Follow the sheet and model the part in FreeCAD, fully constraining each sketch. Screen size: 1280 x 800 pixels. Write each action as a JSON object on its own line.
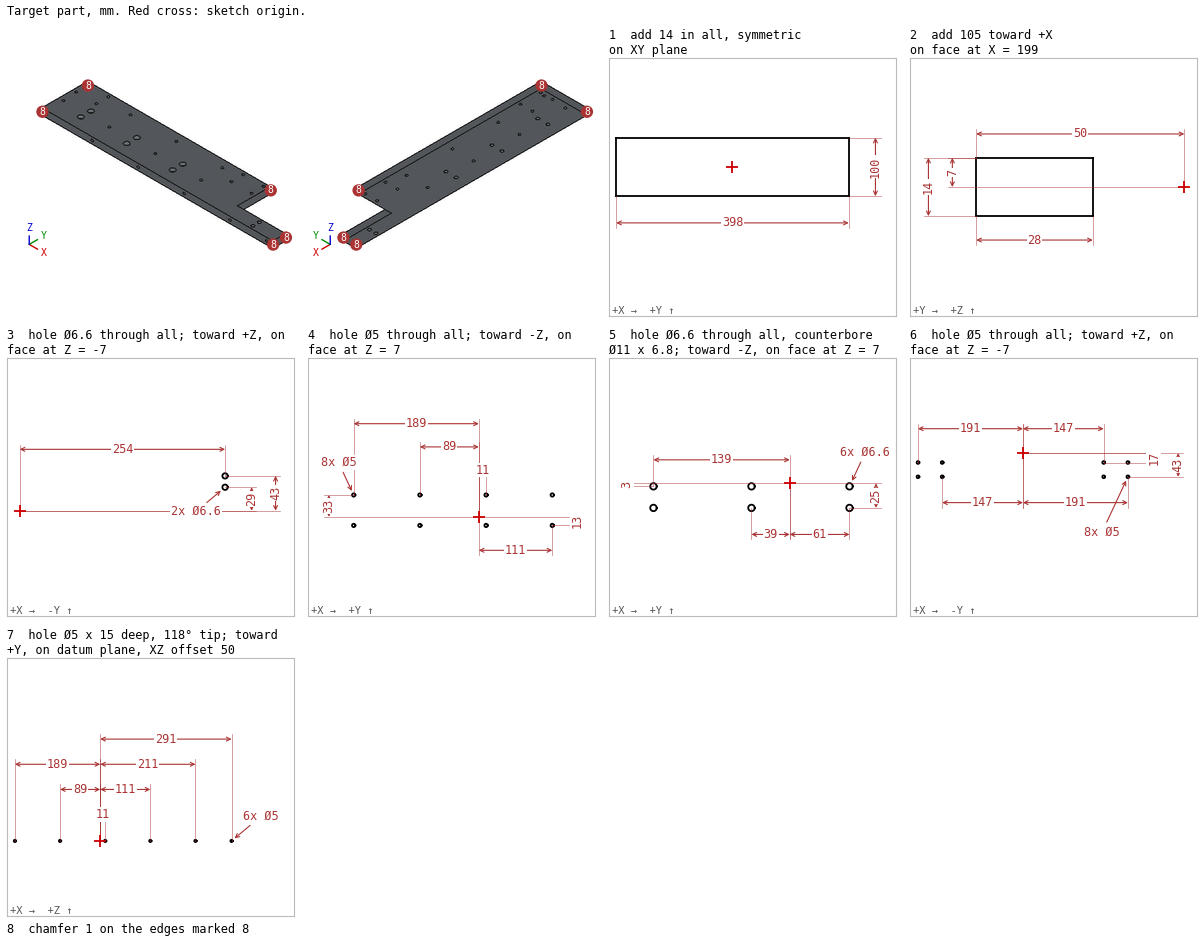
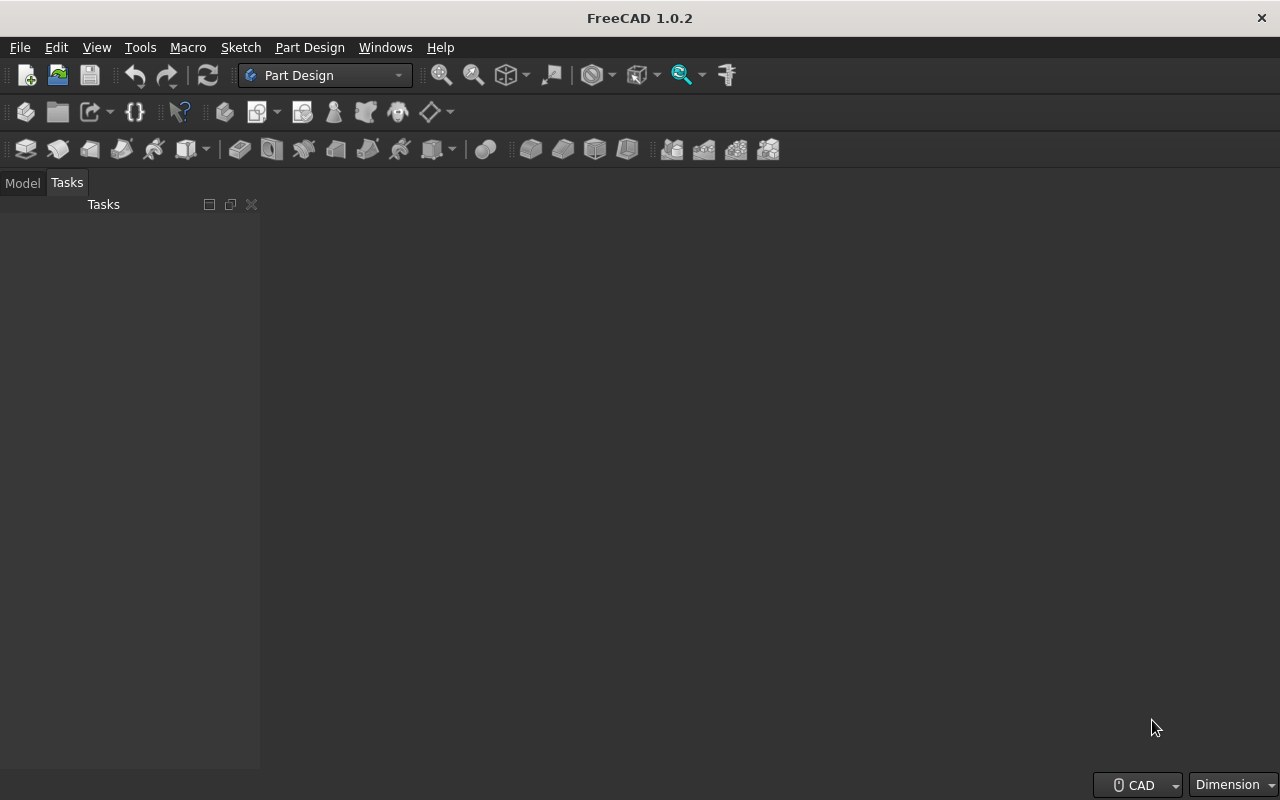
{"action": "key", "text": "ctrl+n"}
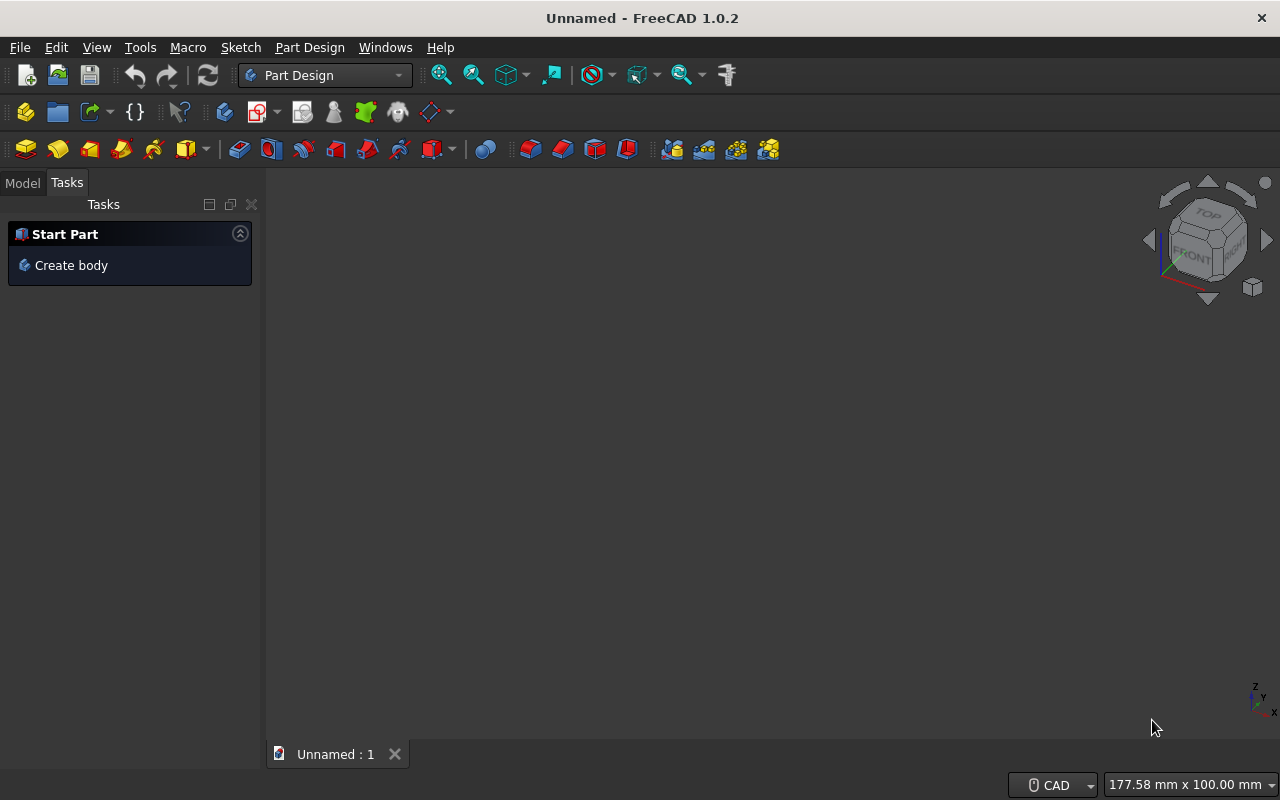
{"action": "left_click", "coordinate": [258, 112]}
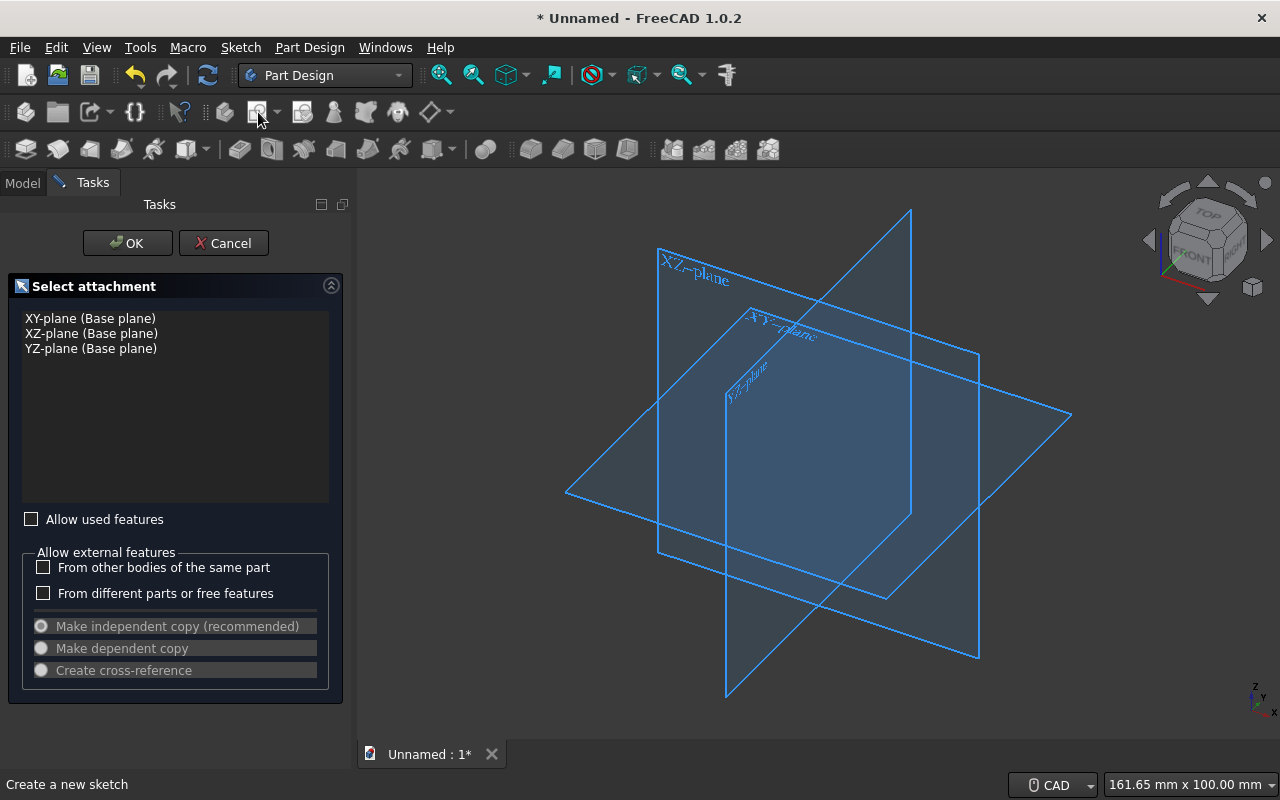
{"action": "left_click", "coordinate": [82, 318]}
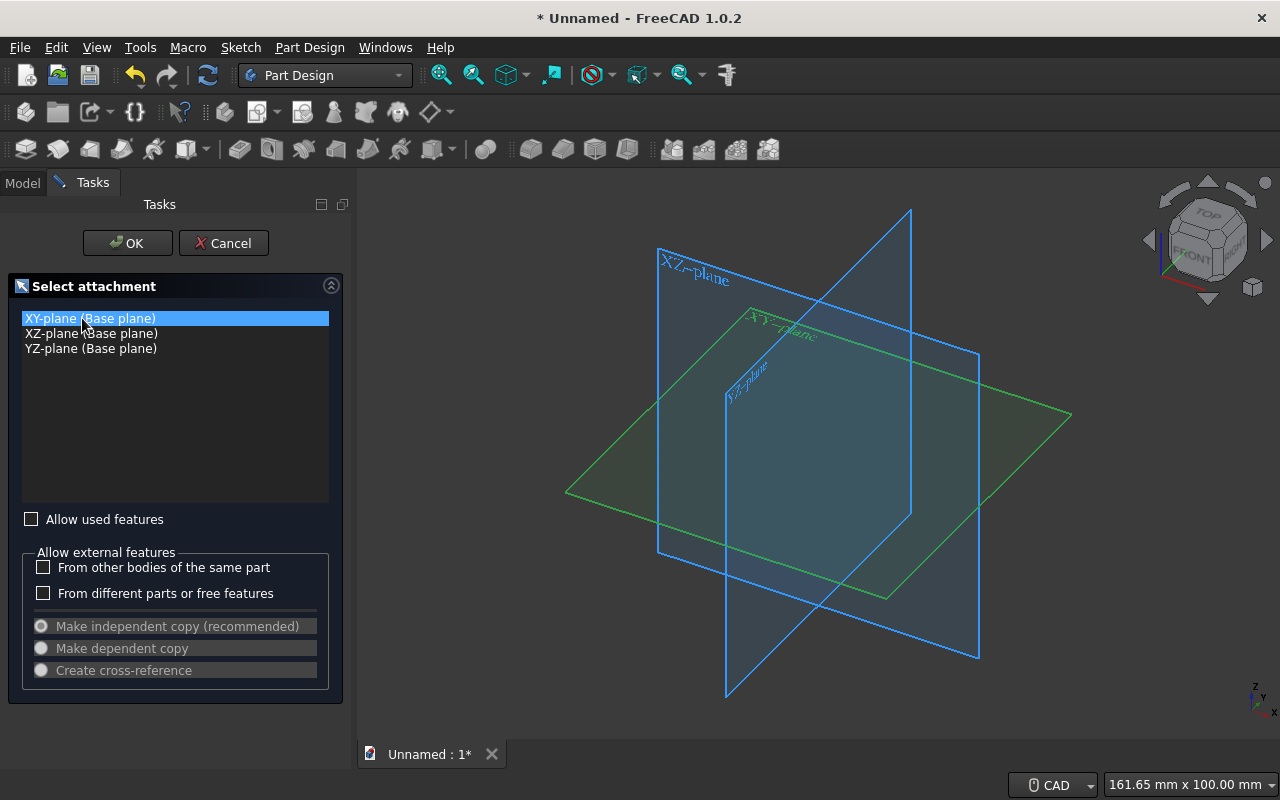
{"action": "left_click", "coordinate": [128, 243]}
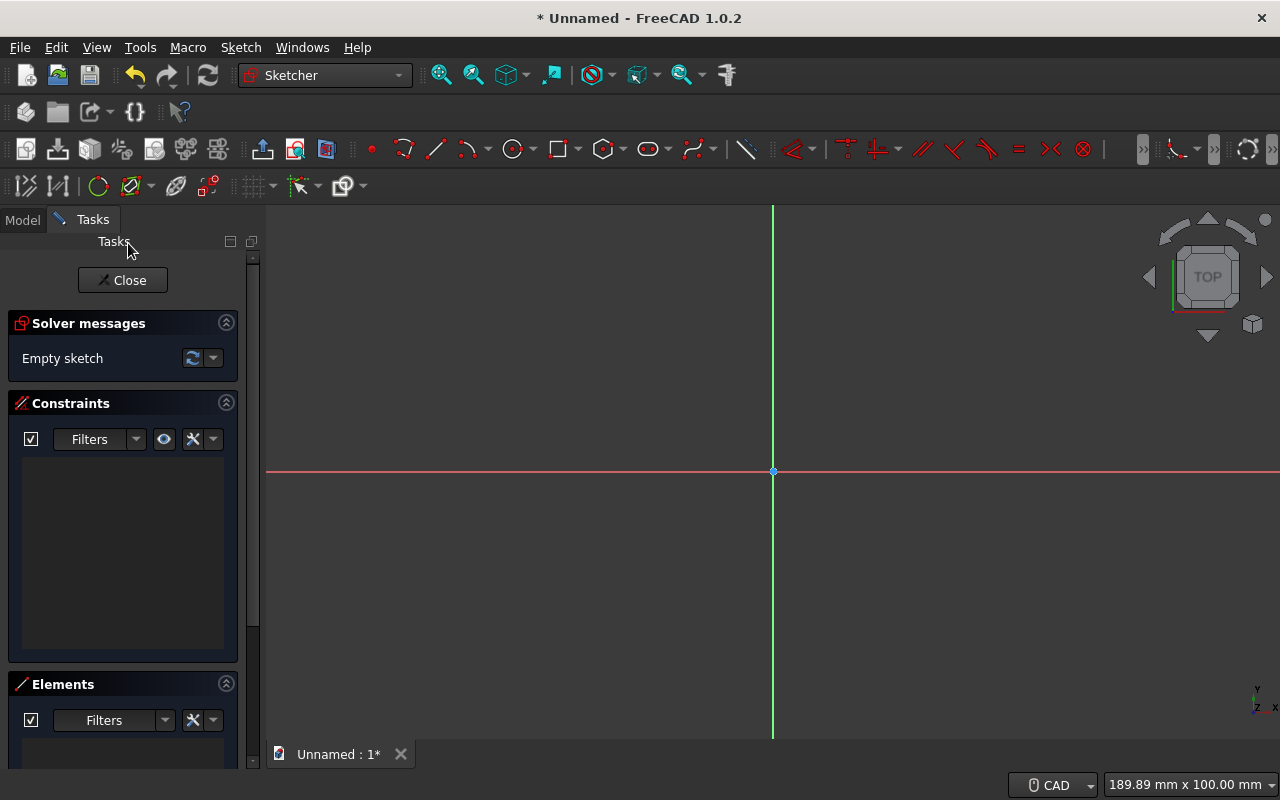
{"action": "scroll", "coordinate": [675, 472], "scroll_direction": "down", "scroll_amount": 6}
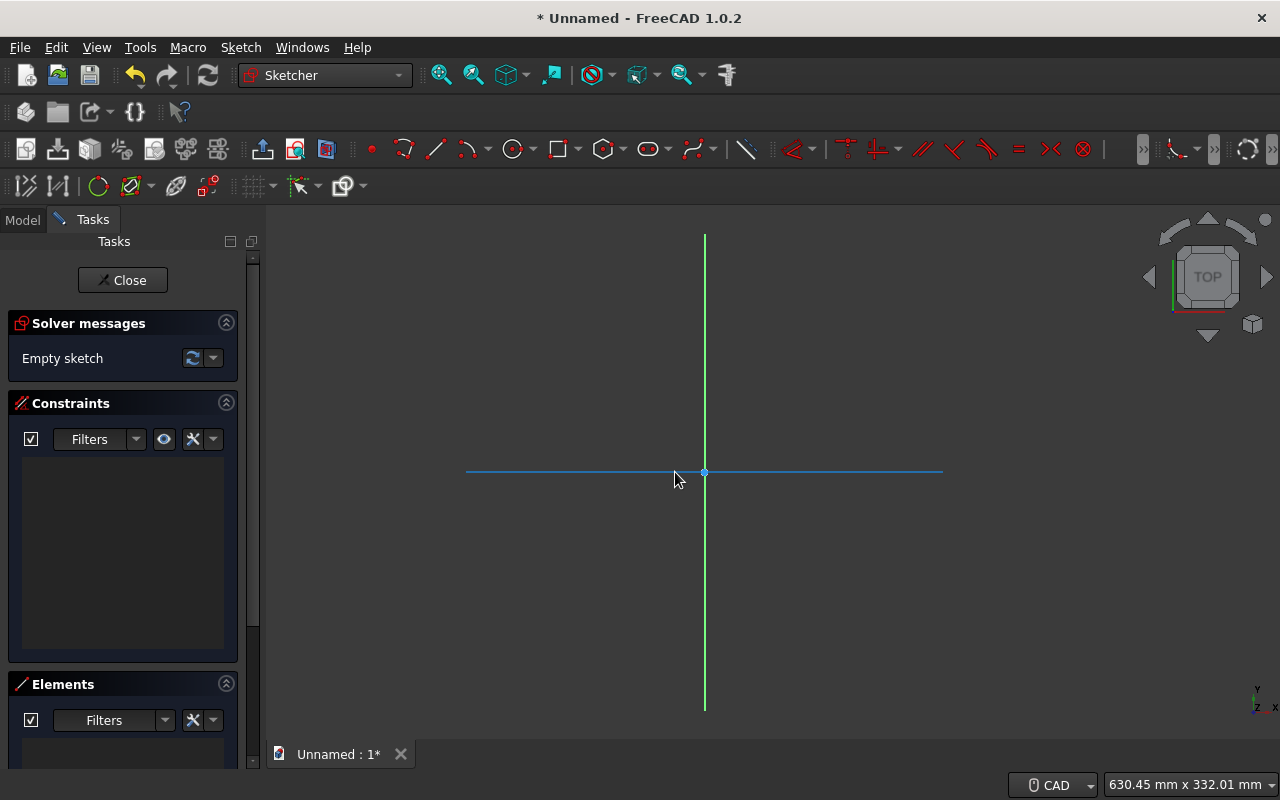
{"action": "key", "text": "g v"}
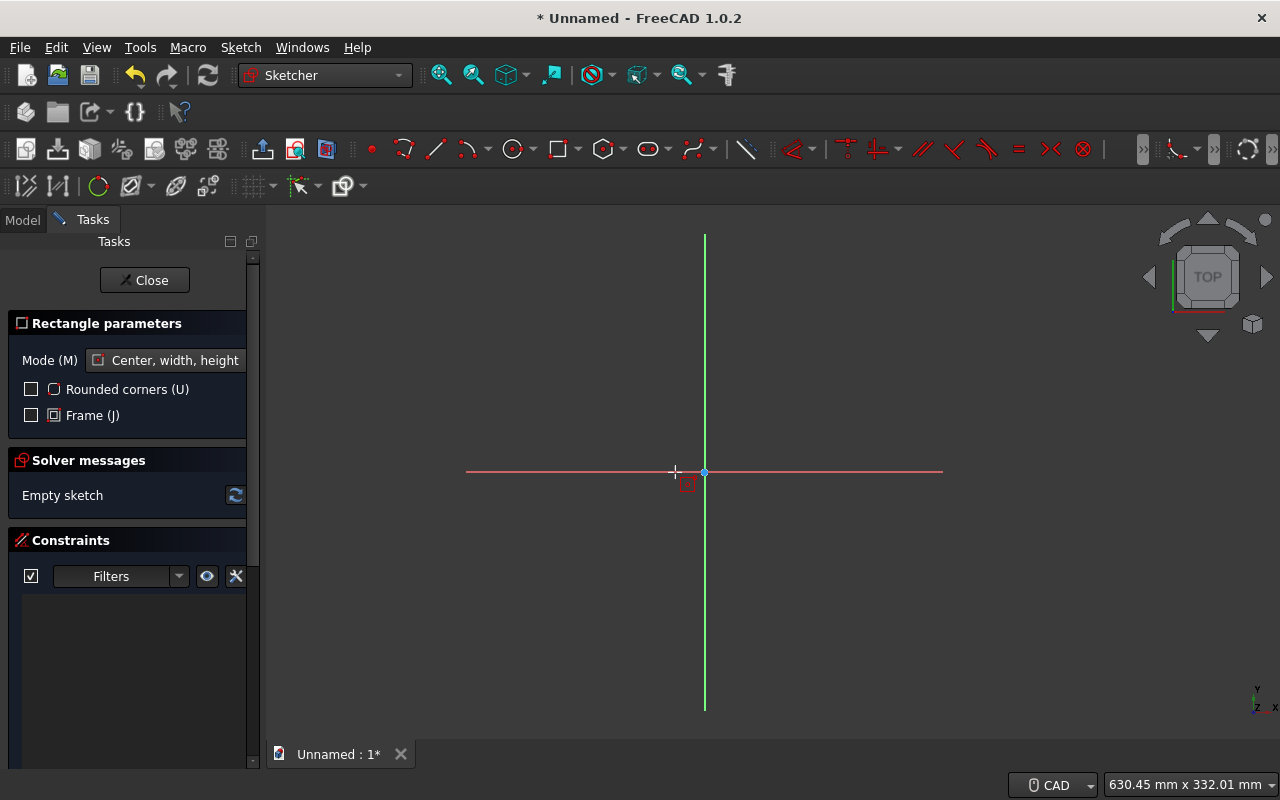
{"action": "left_click", "coordinate": [705, 472]}
{"action": "left_click", "coordinate": [1025, 392]}
{"action": "key", "text": "Escape"}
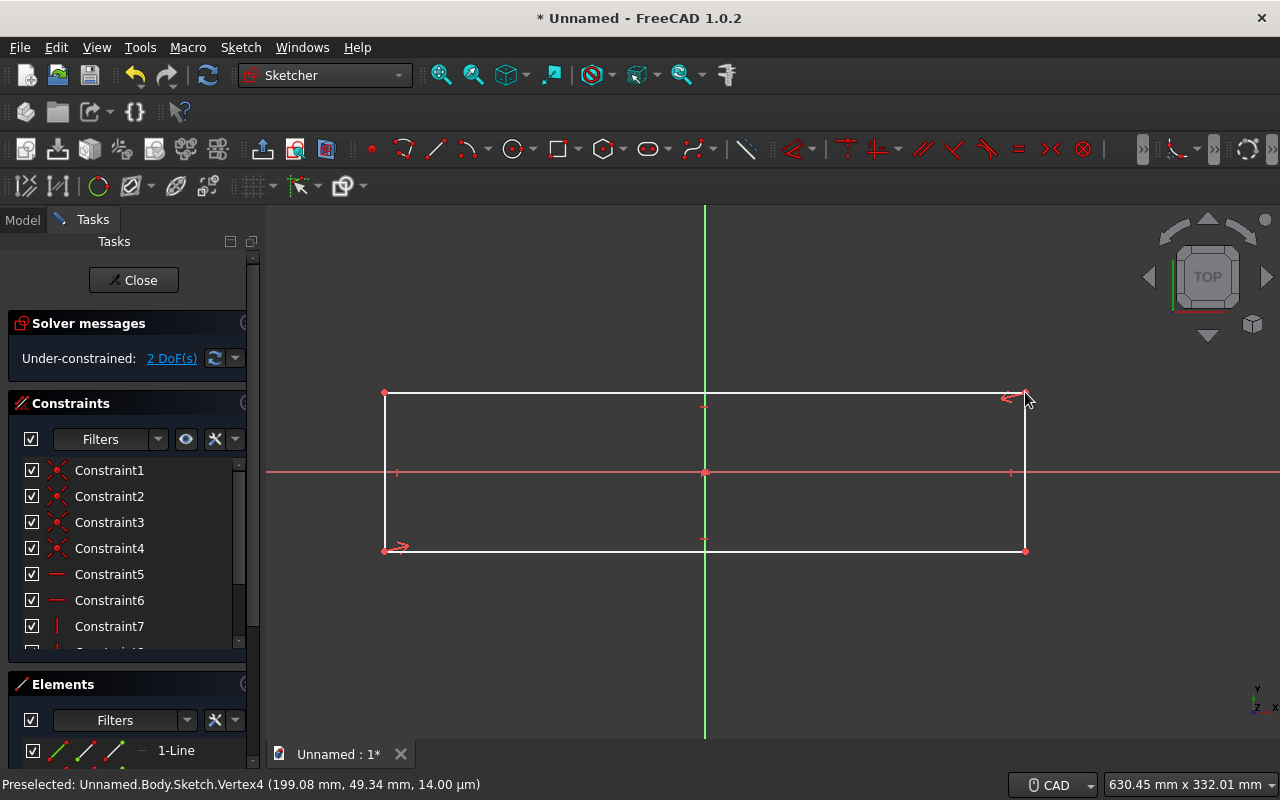
{"action": "left_click", "coordinate": [792, 150]}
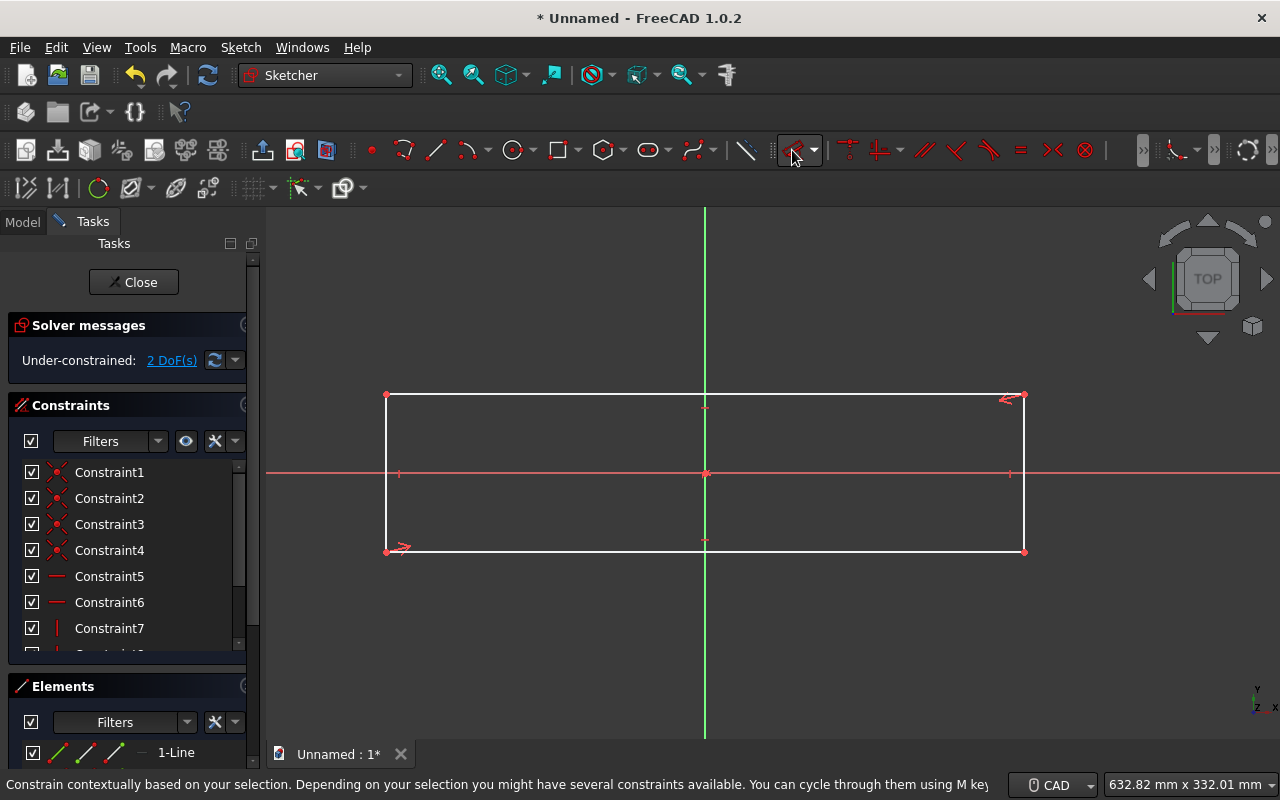
{"action": "left_click", "coordinate": [577, 552]}
{"action": "left_click", "coordinate": [558, 586]}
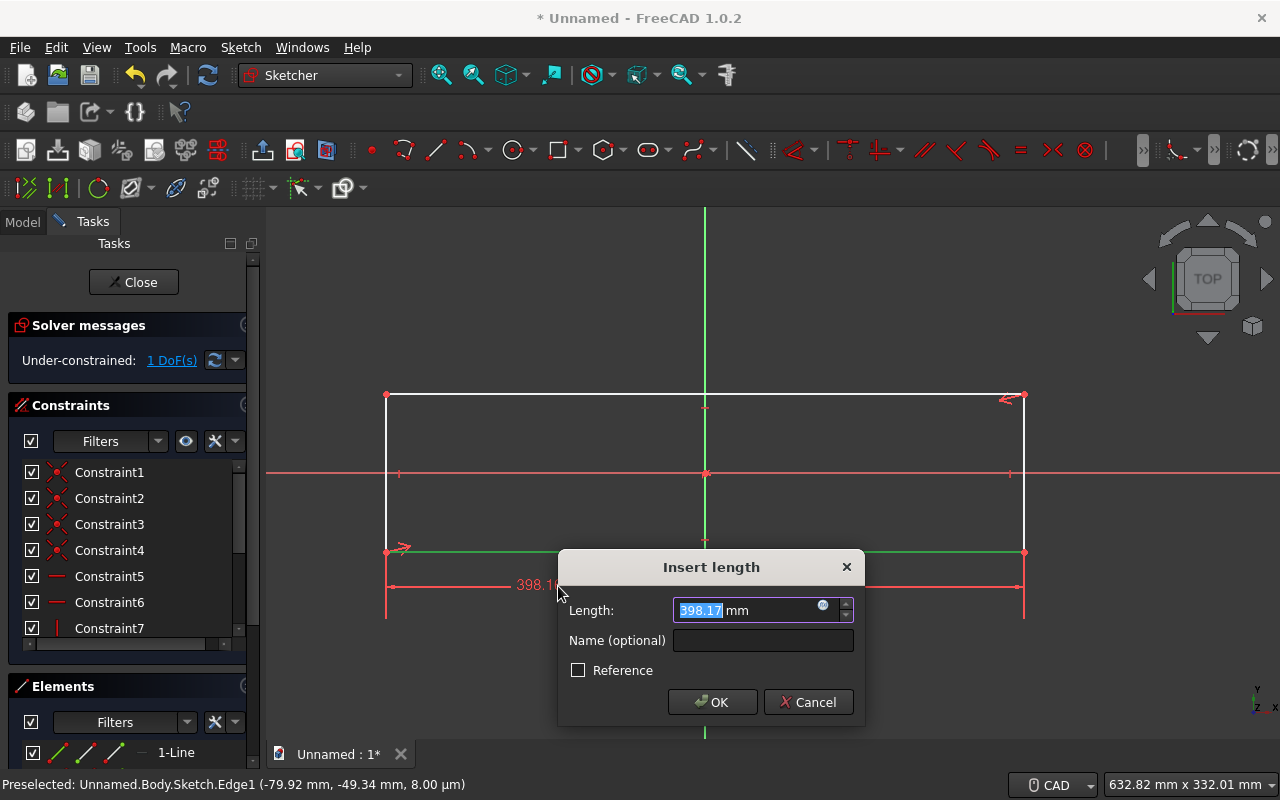
{"action": "type", "text": "398"}
{"action": "key", "text": "Return"}